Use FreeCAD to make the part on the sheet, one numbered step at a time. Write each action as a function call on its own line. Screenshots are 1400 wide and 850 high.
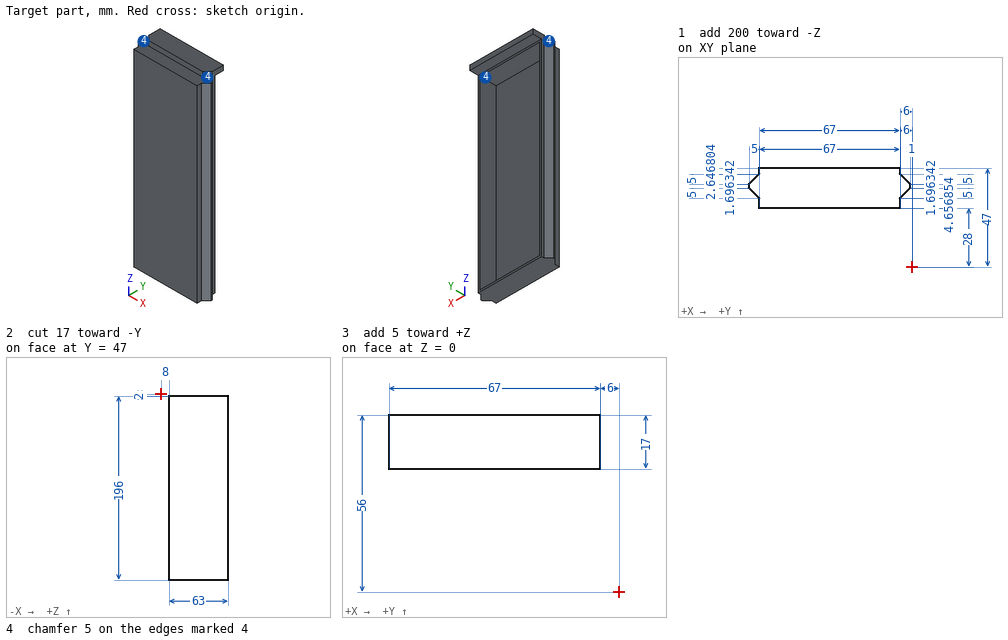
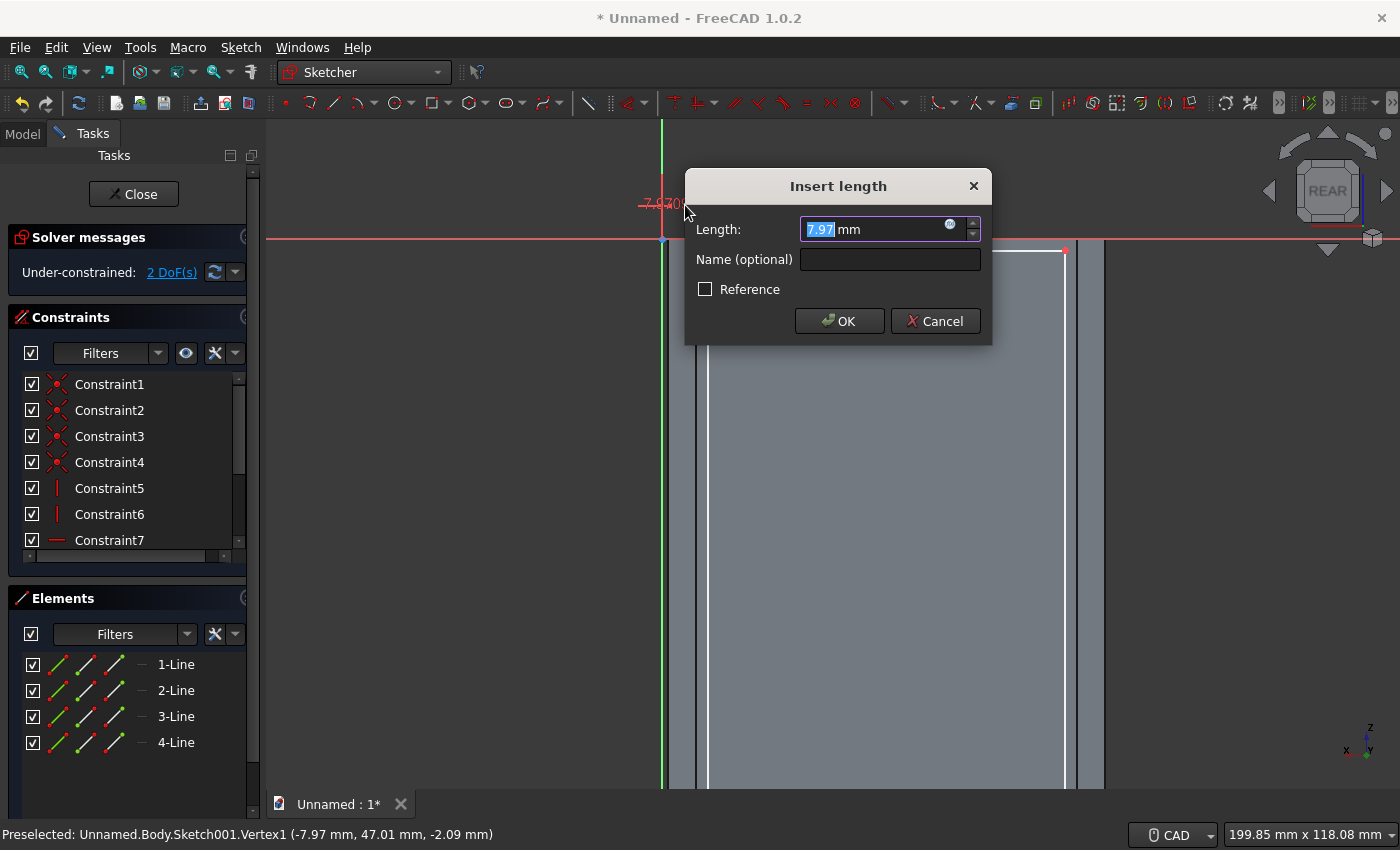
text(8)
key(Return)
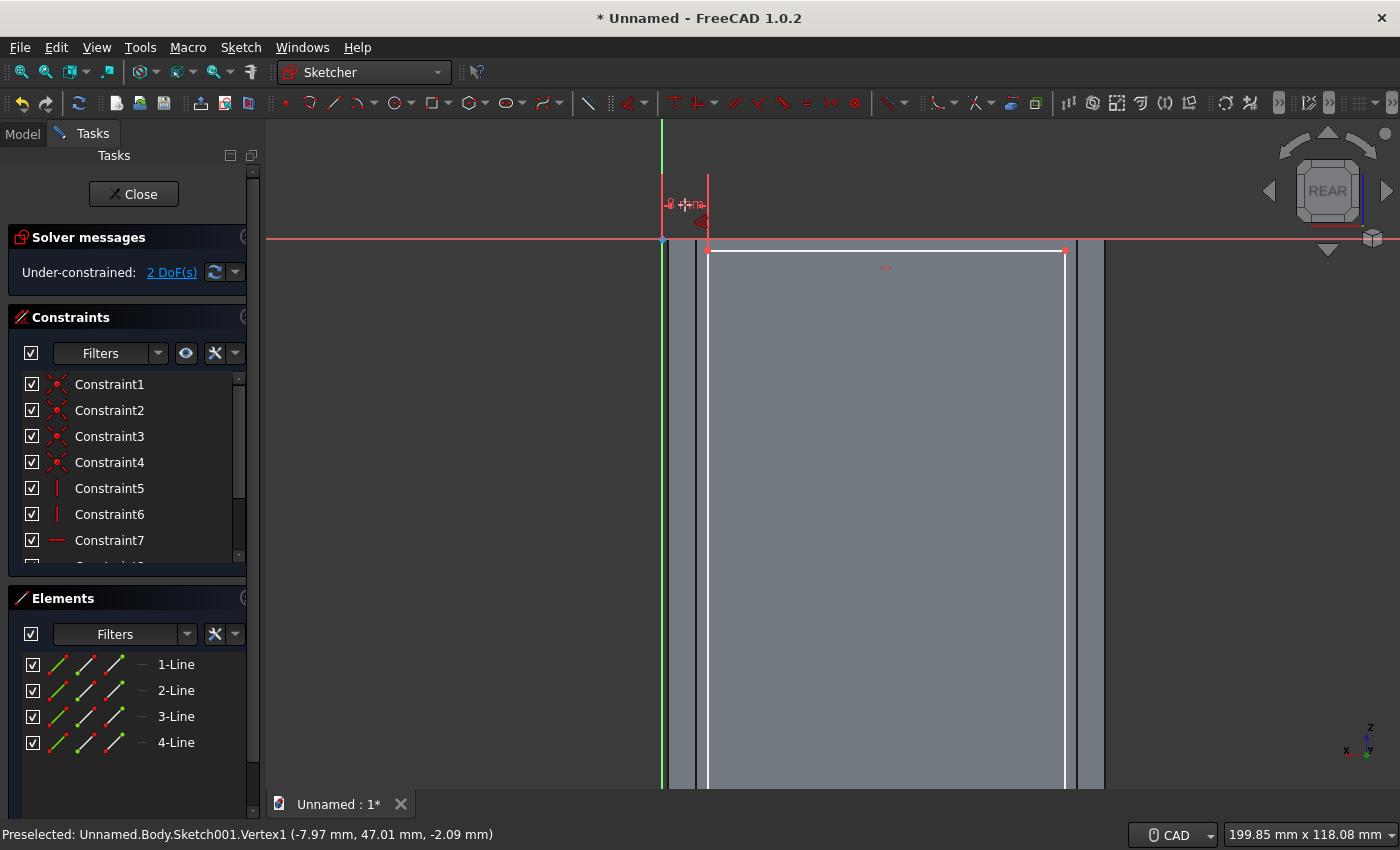
scroll(708, 251, up, 7)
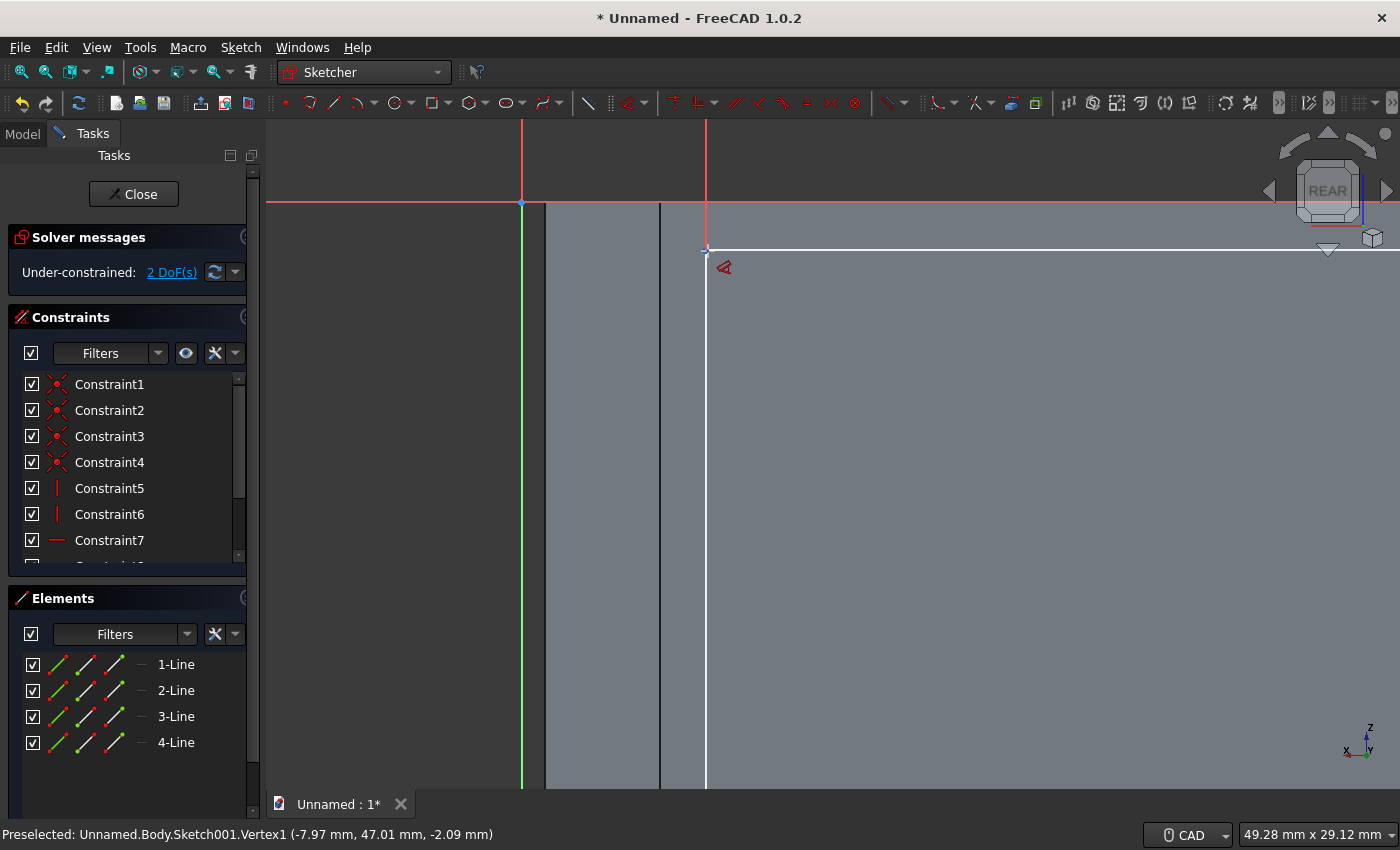
click(706, 250)
click(488, 226)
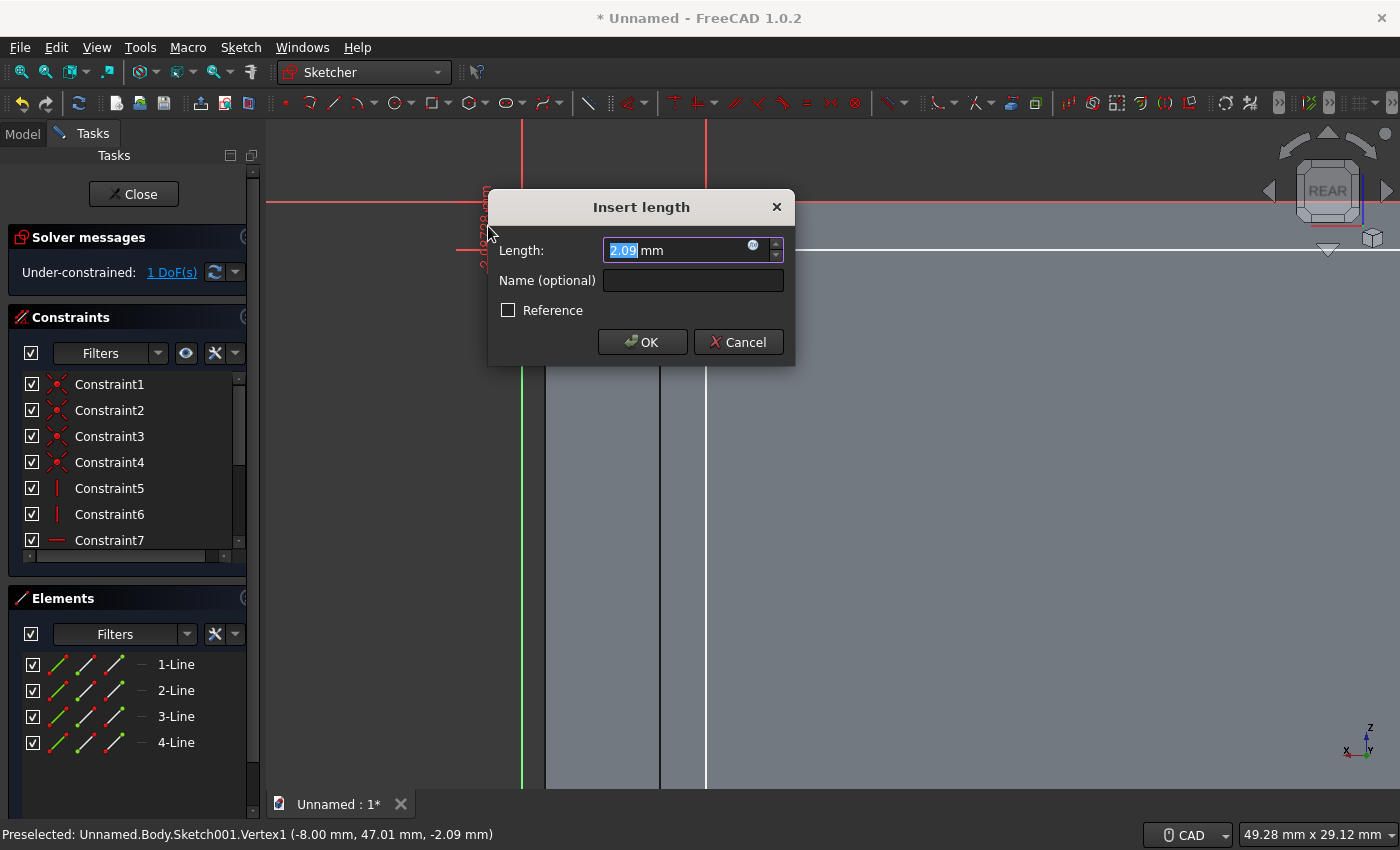
text(2)
key(Return)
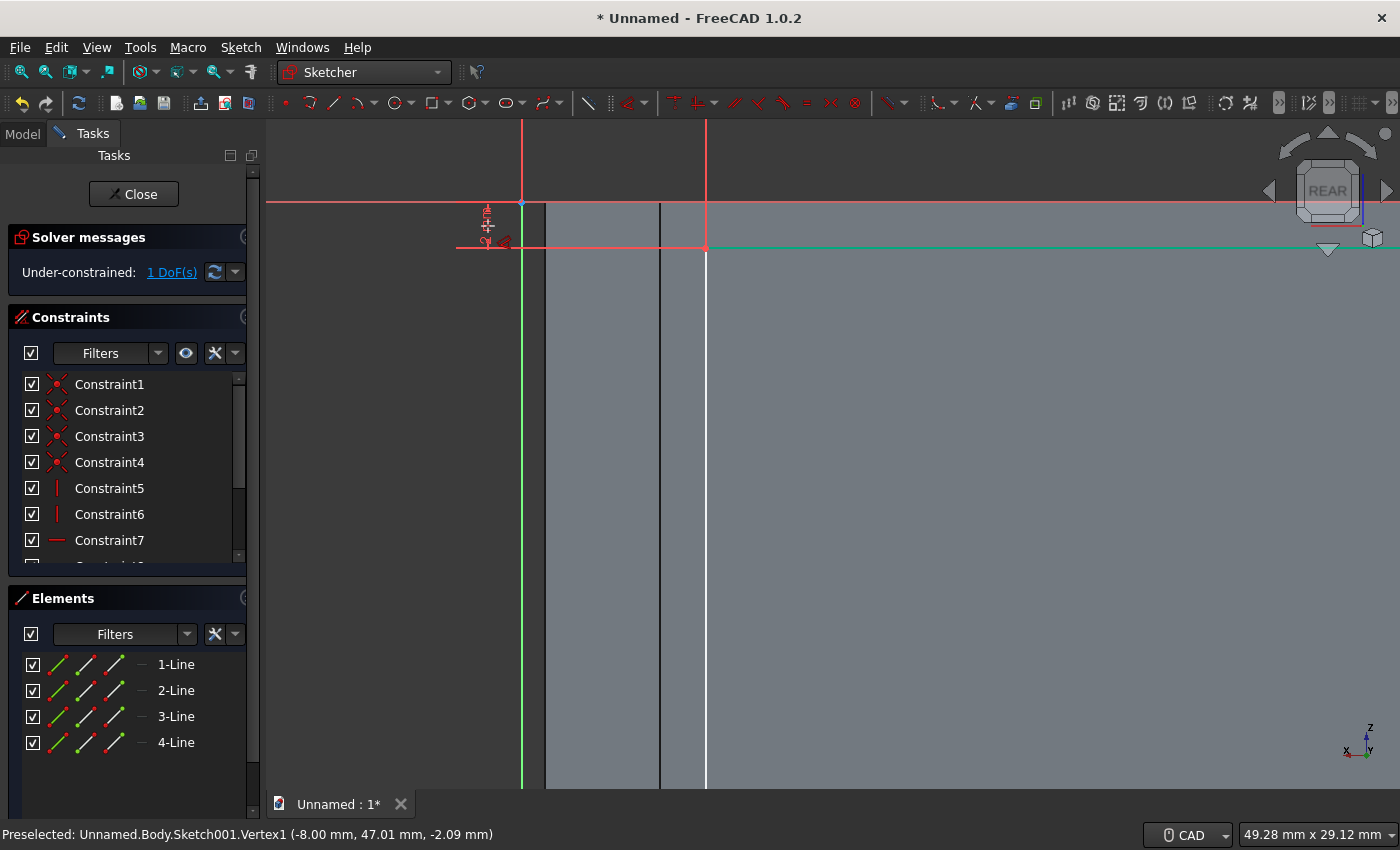
scroll(707, 252, down, 12)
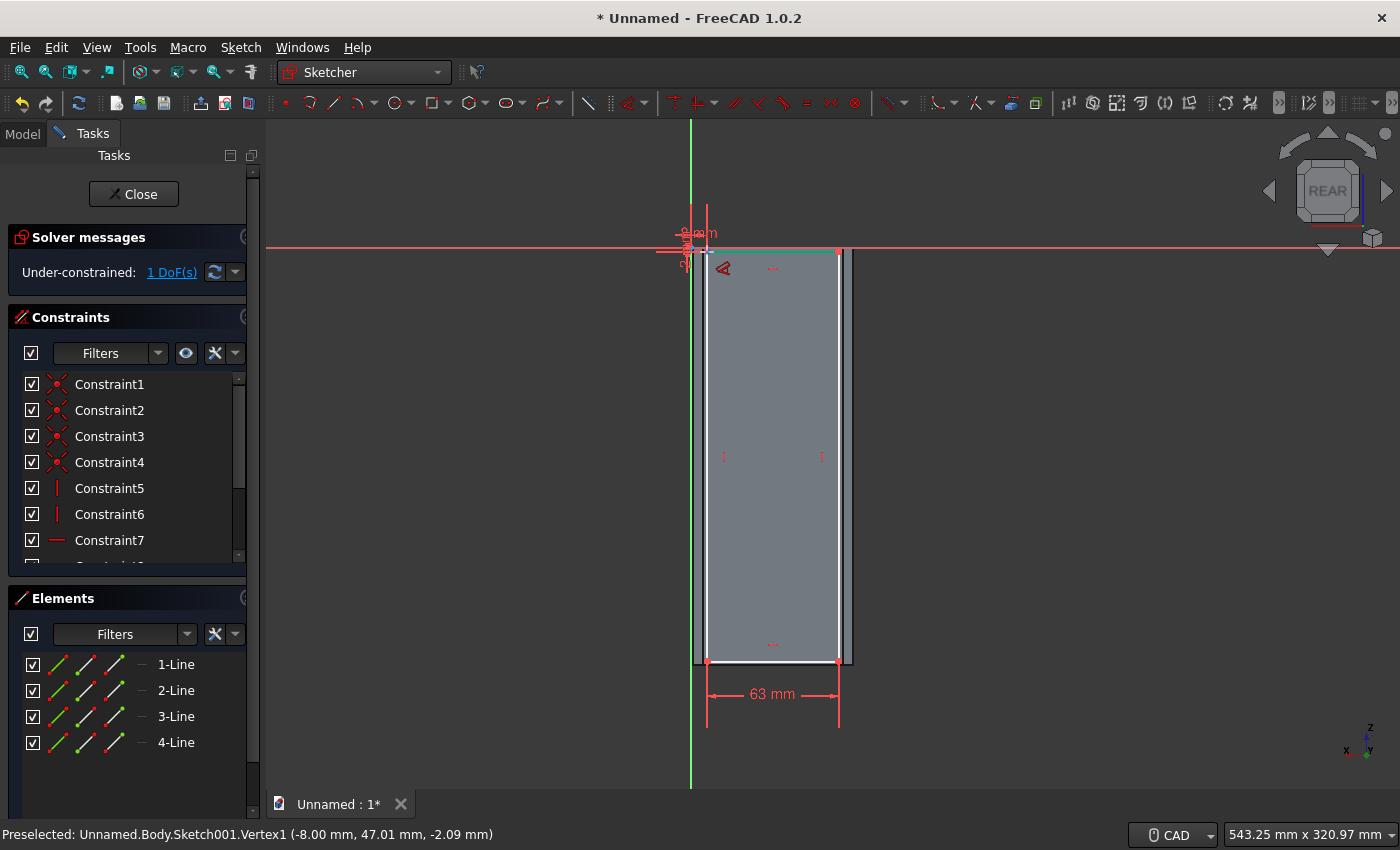
click(707, 375)
click(673, 457)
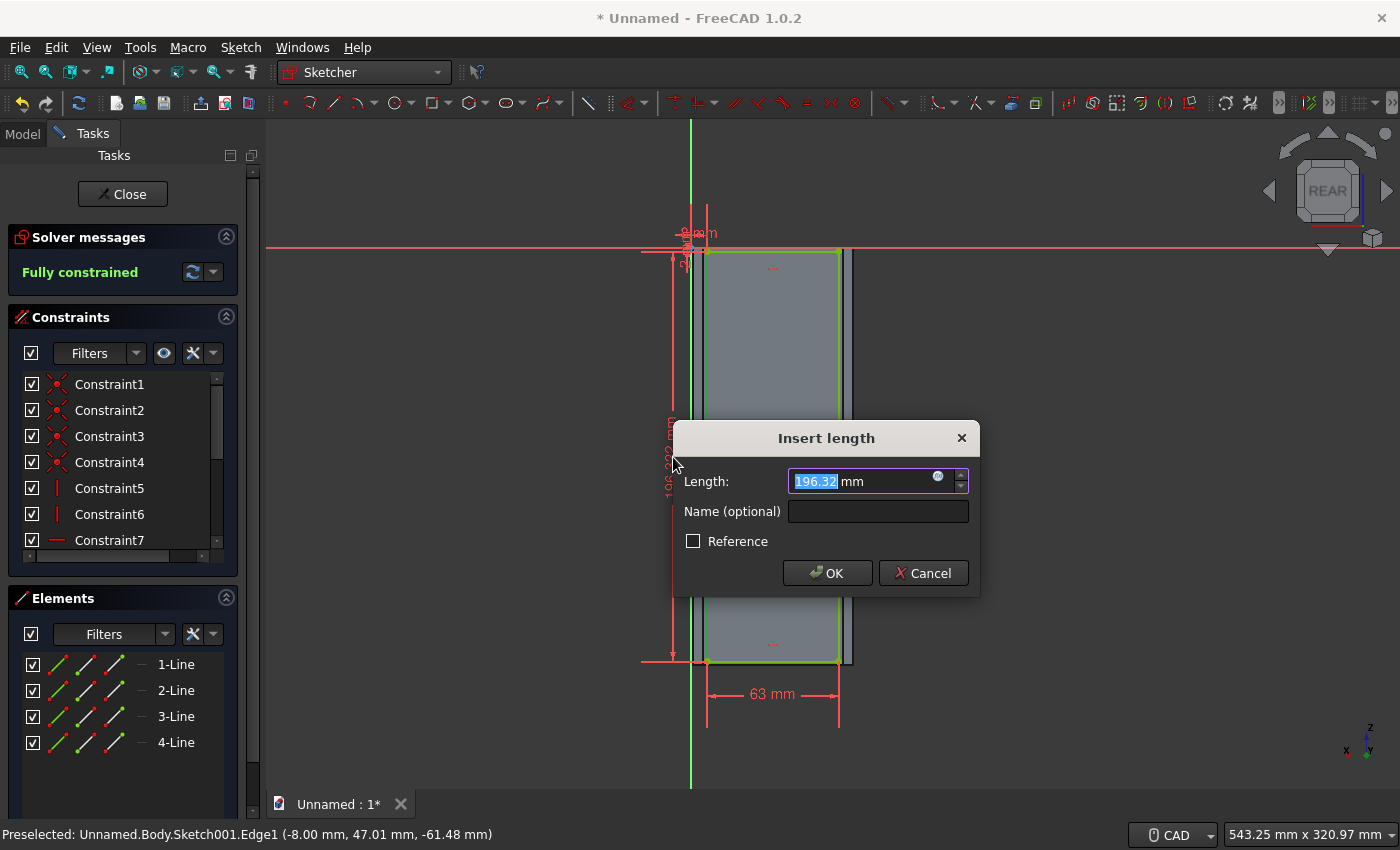
text(196)
key(Return)
key(Escape)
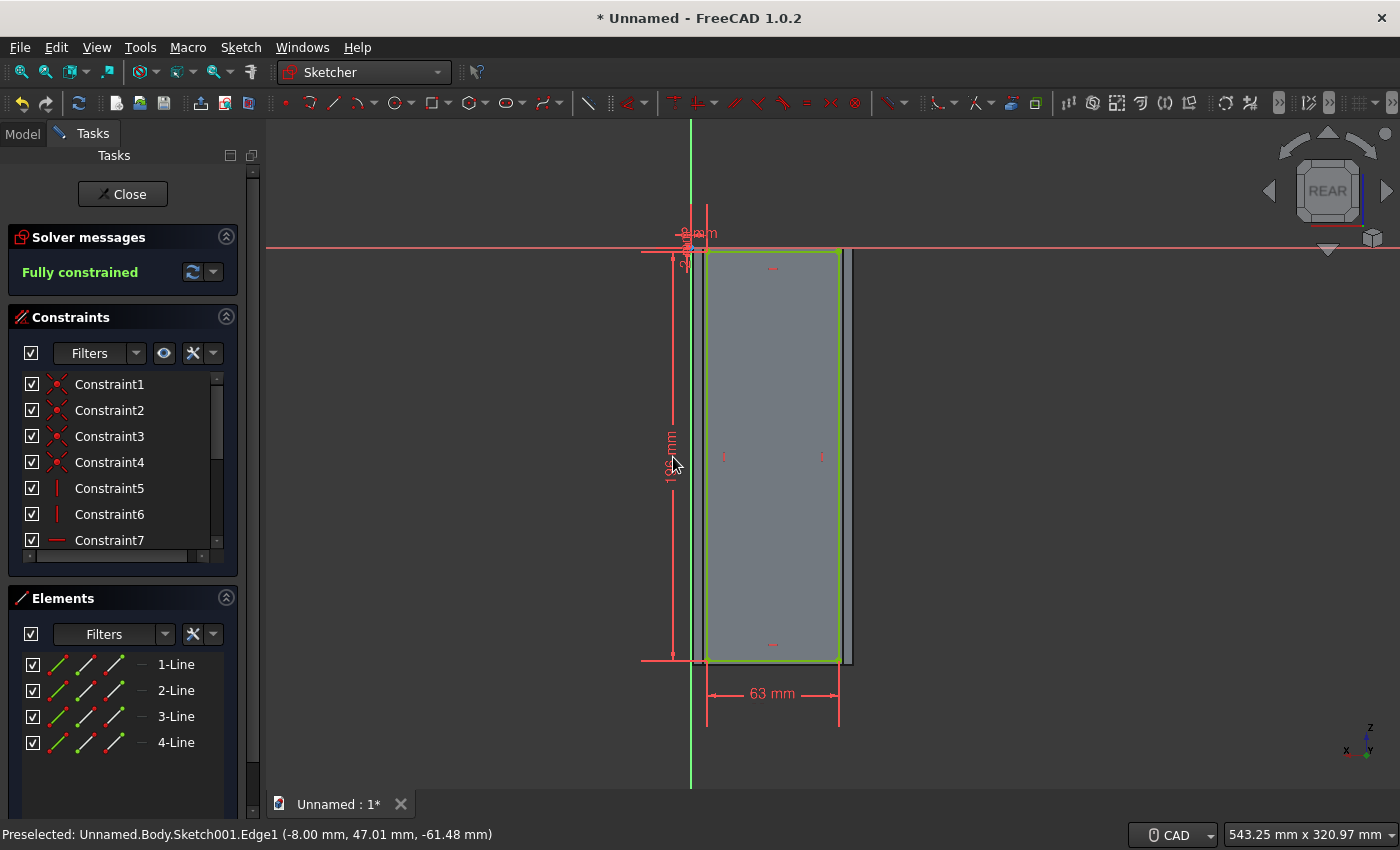
click(123, 194)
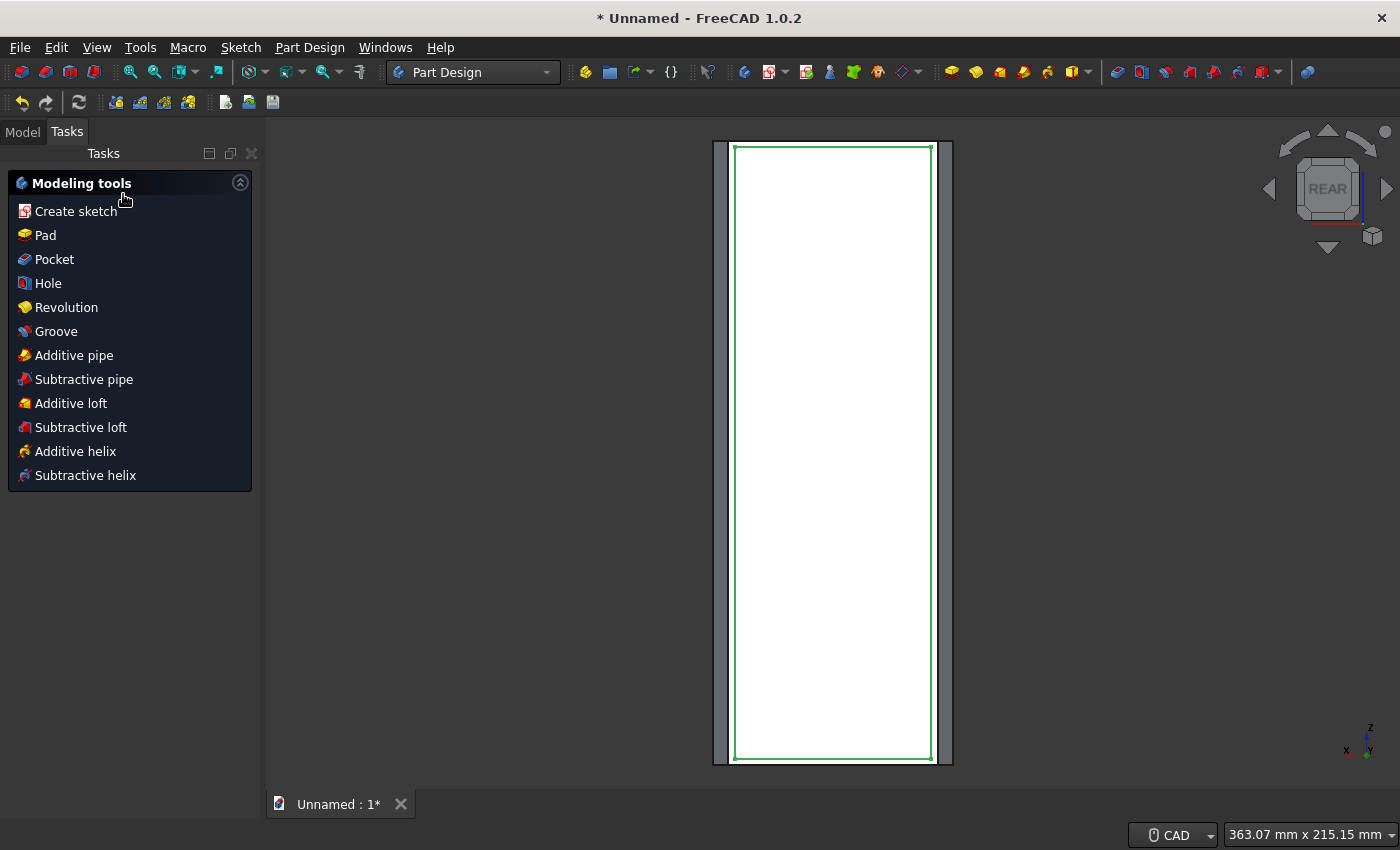
click(1118, 72)